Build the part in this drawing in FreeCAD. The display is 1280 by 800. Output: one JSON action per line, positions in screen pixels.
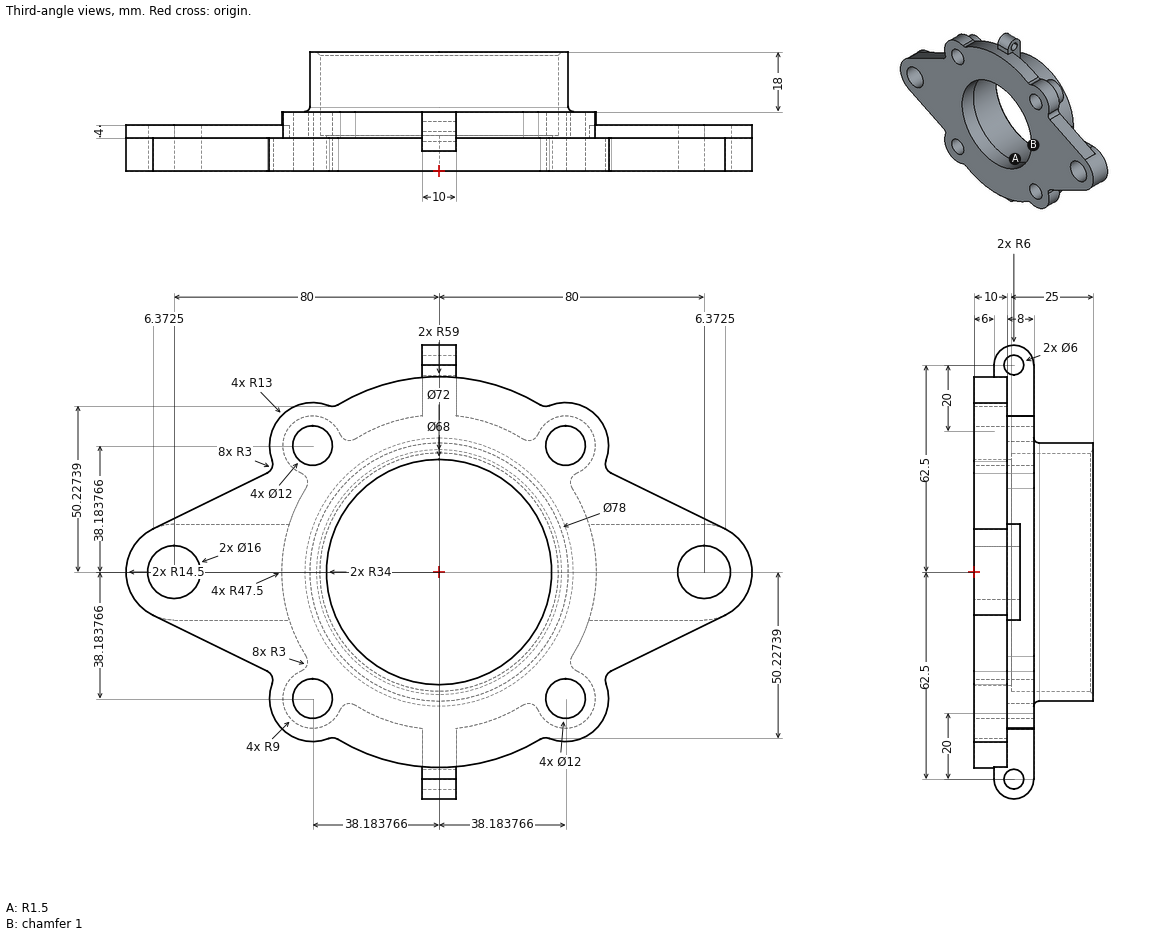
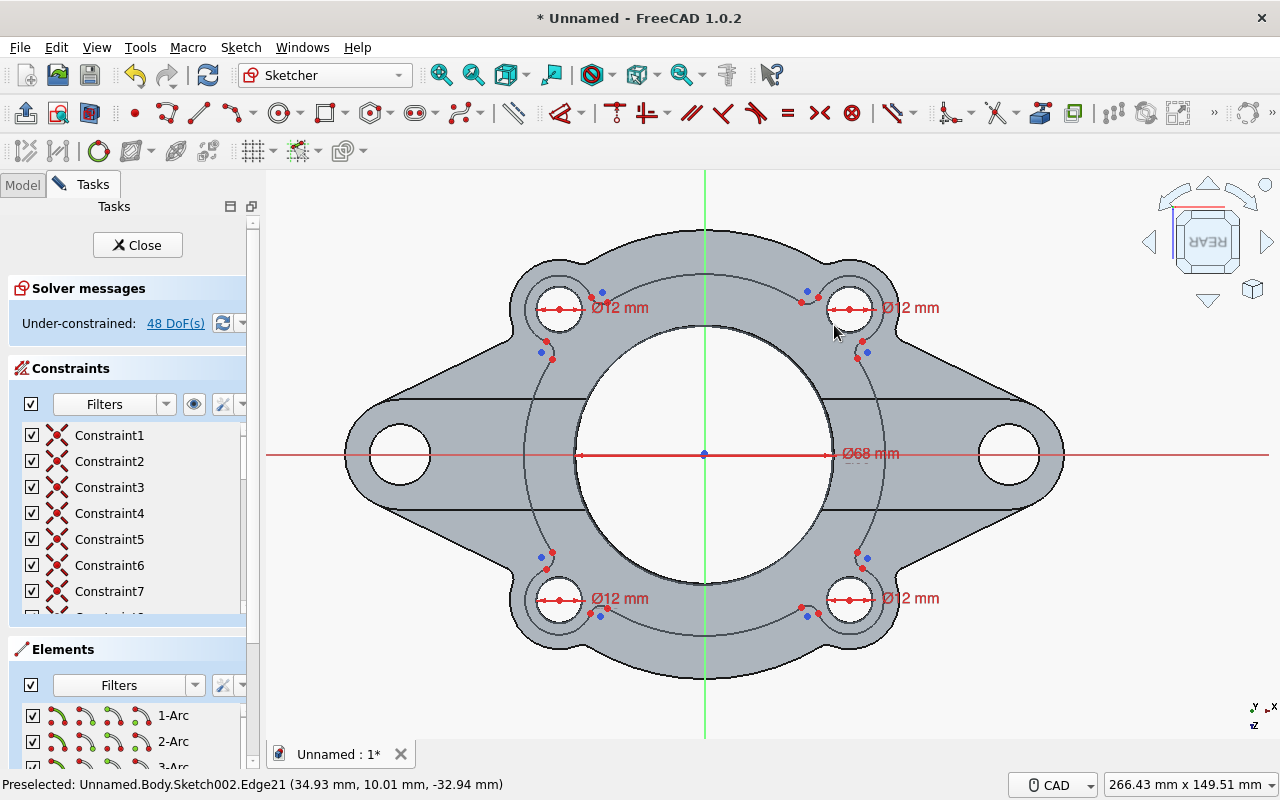
{"action": "left_click", "coordinate": [529, 415]}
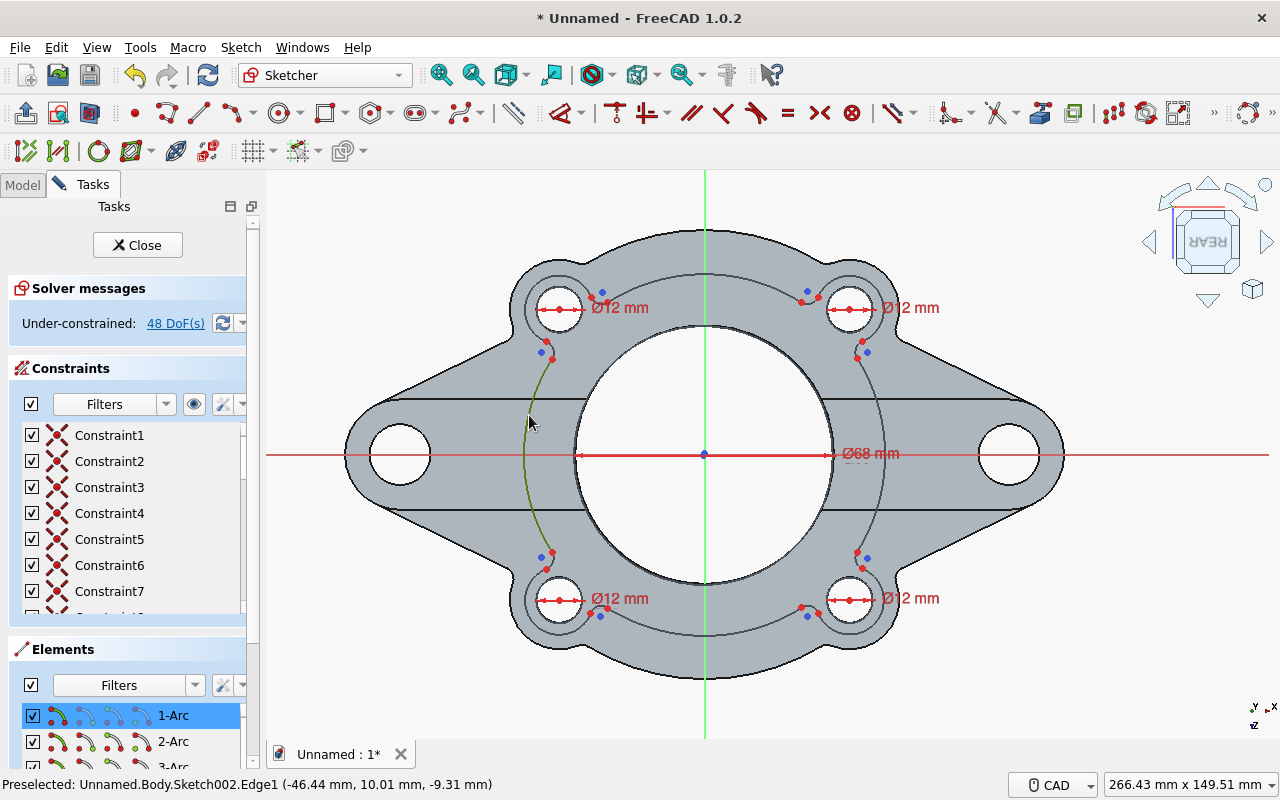
{"action": "scroll", "coordinate": [553, 562], "scroll_direction": "up", "scroll_amount": 2}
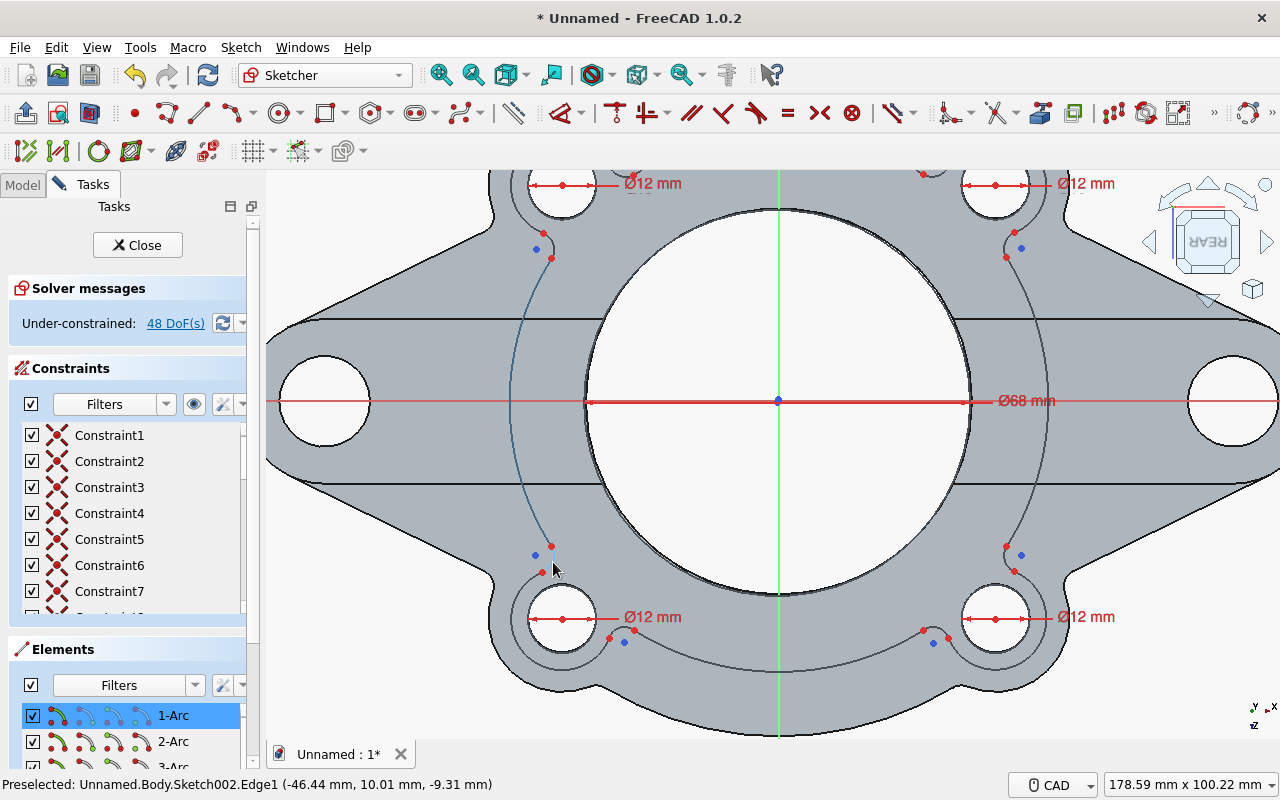
{"action": "left_click", "coordinate": [553, 562]}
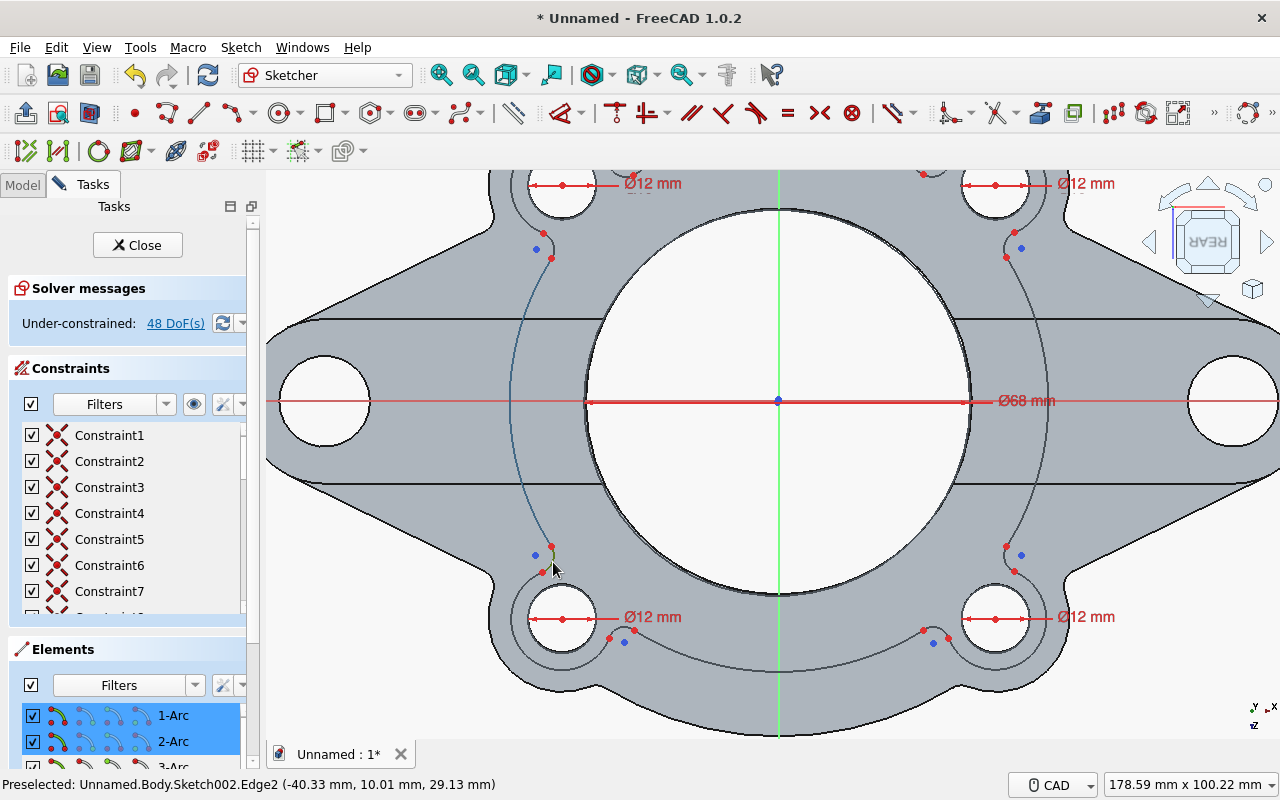
{"action": "left_click", "coordinate": [756, 114]}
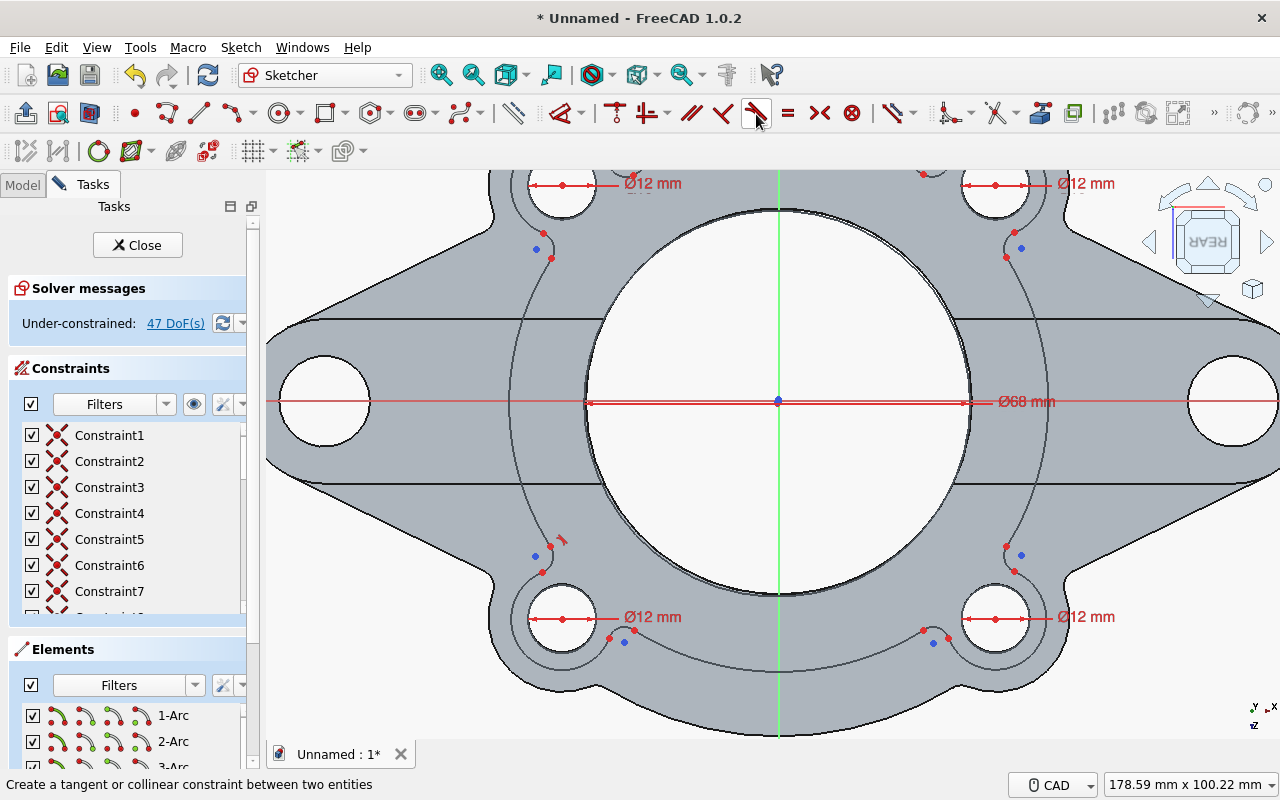
{"action": "left_click", "coordinate": [516, 342]}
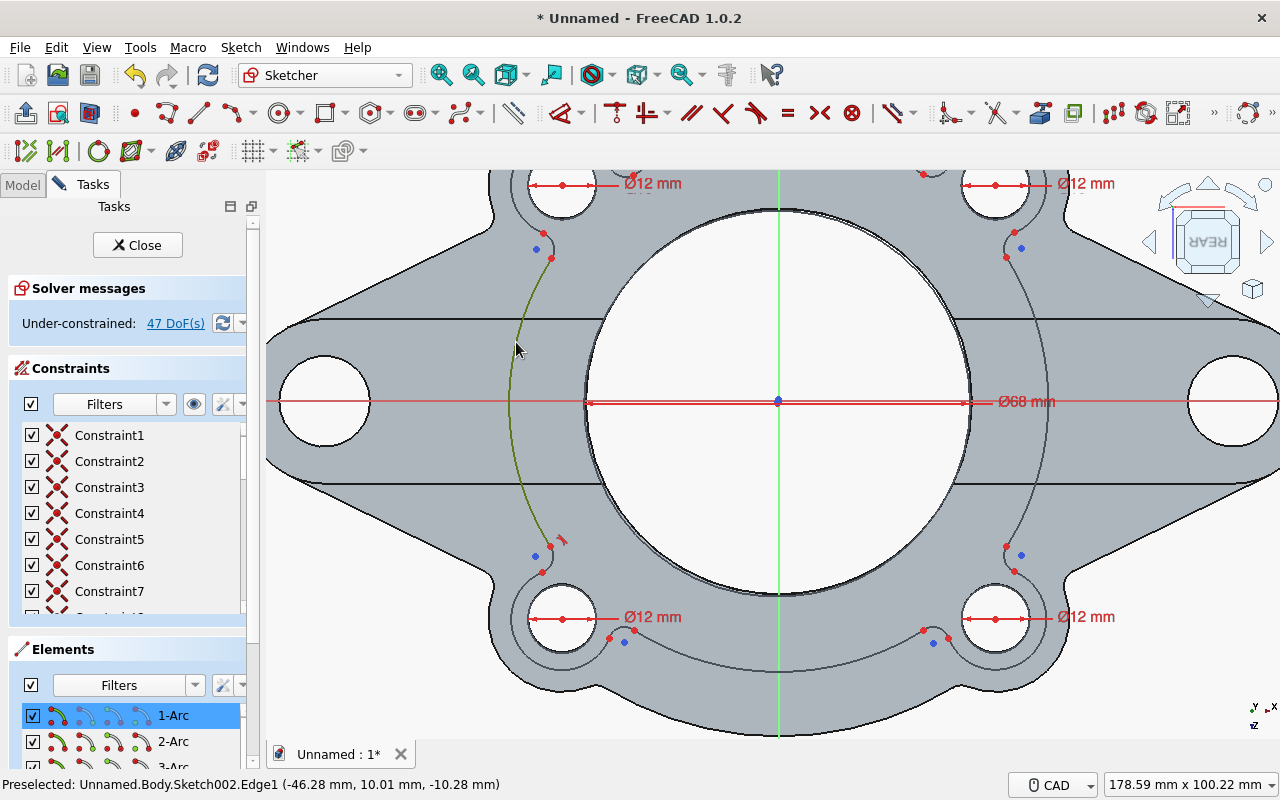
{"action": "scroll", "coordinate": [554, 250], "scroll_direction": "up", "scroll_amount": 3}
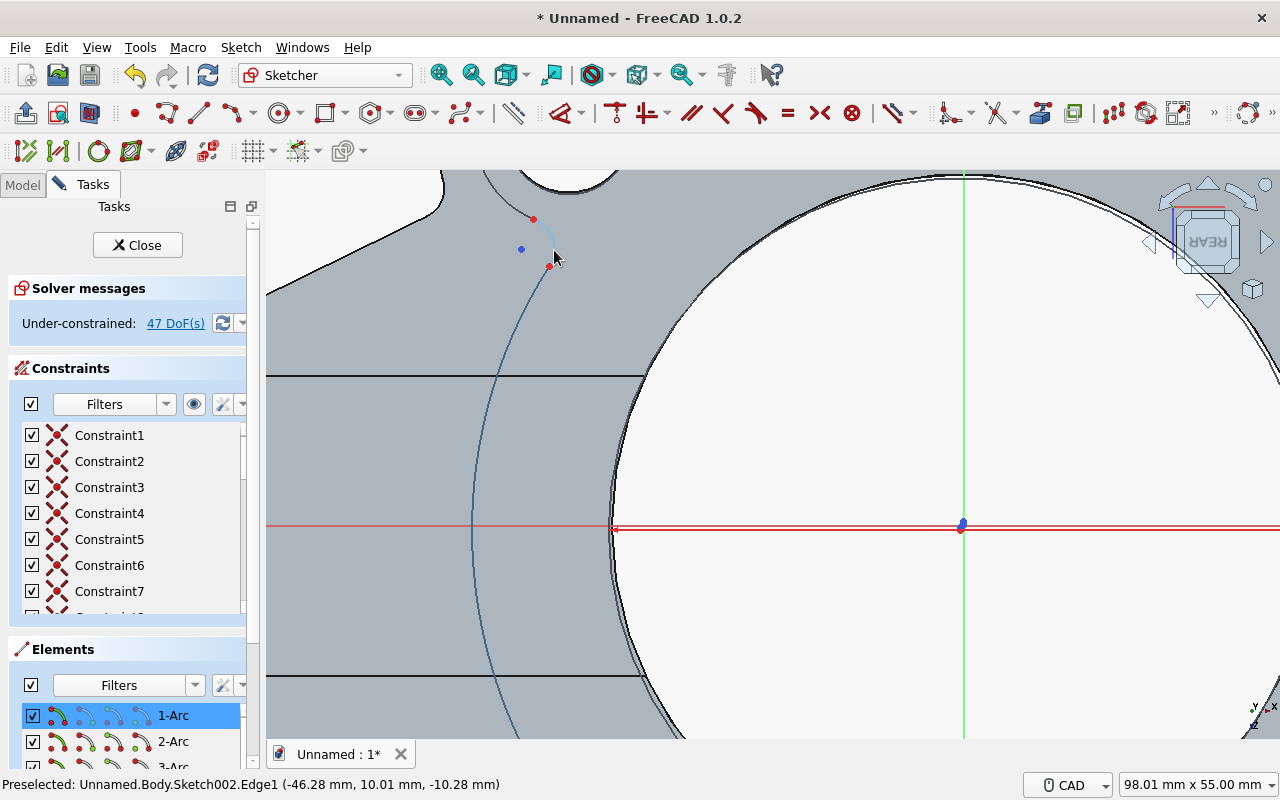
{"action": "left_click", "coordinate": [554, 250]}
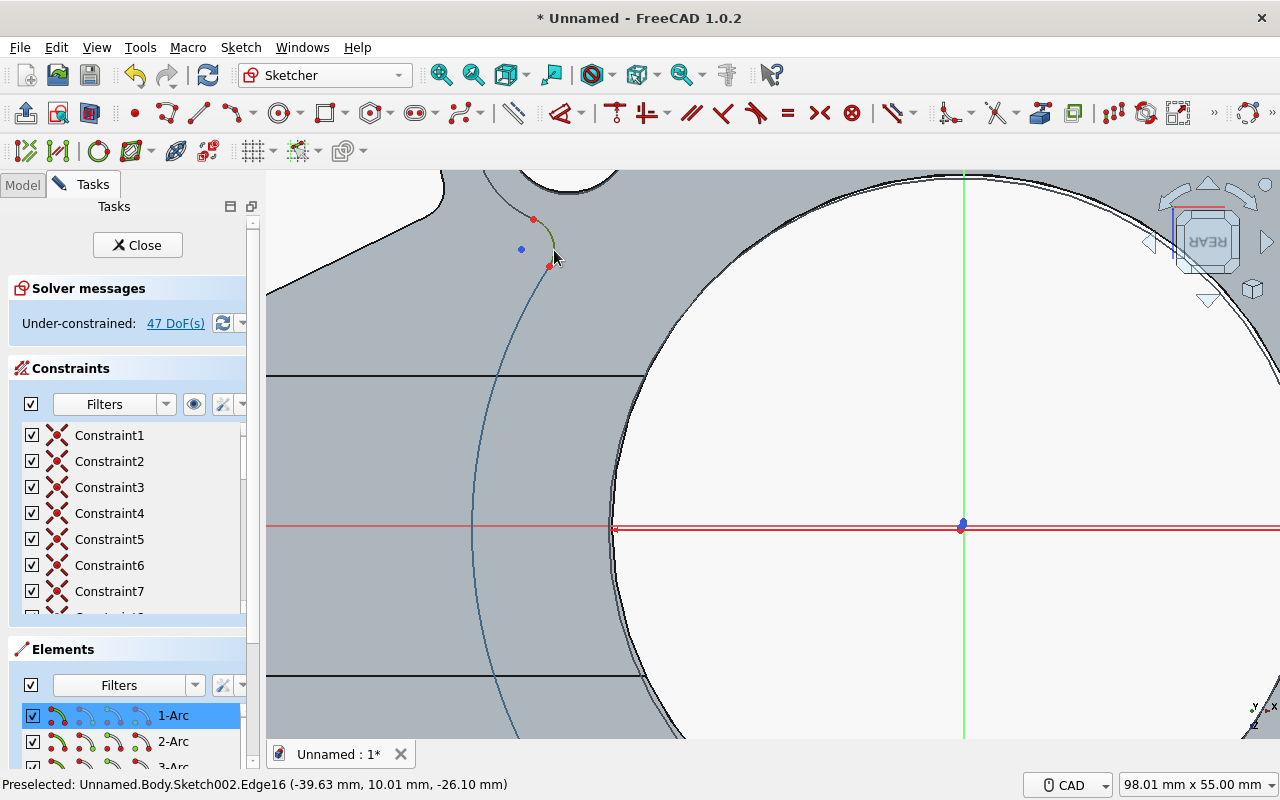
{"action": "left_click", "coordinate": [756, 114]}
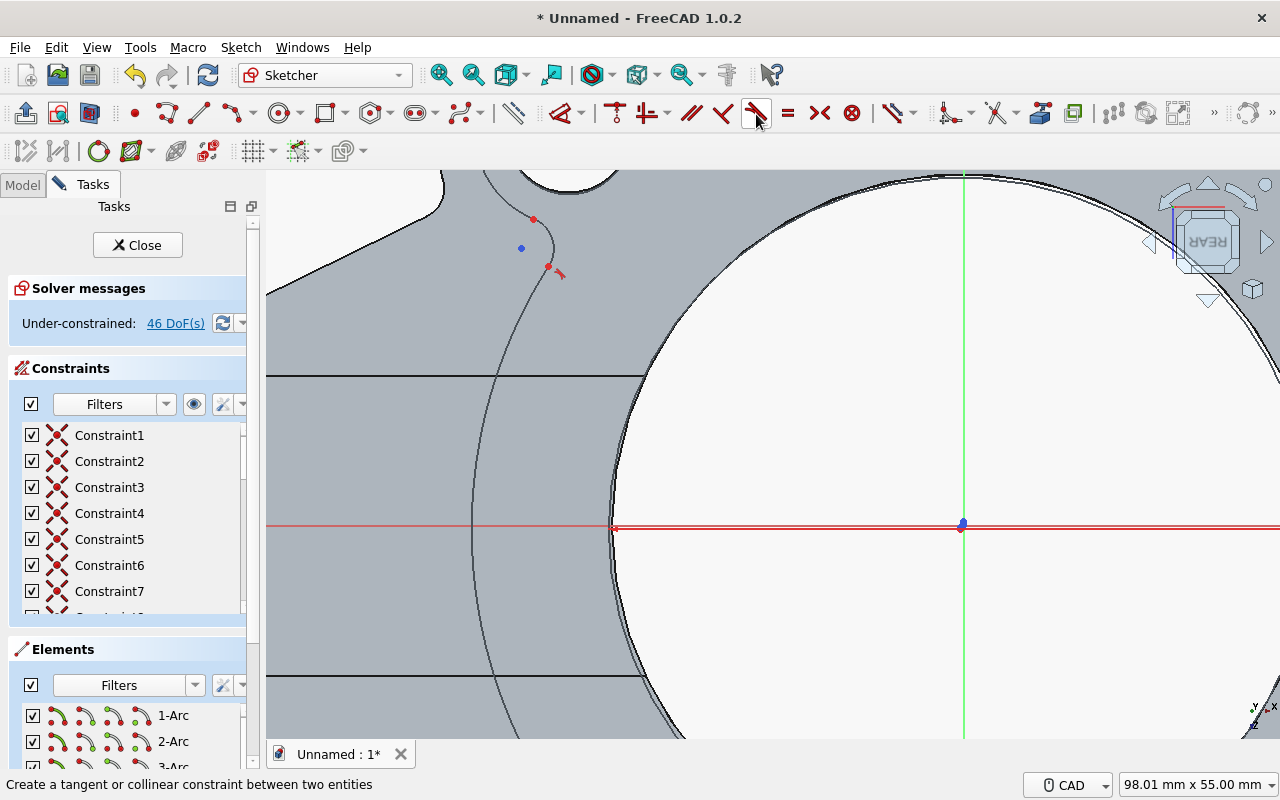
{"action": "scroll", "coordinate": [554, 413], "scroll_direction": "down", "scroll_amount": 5}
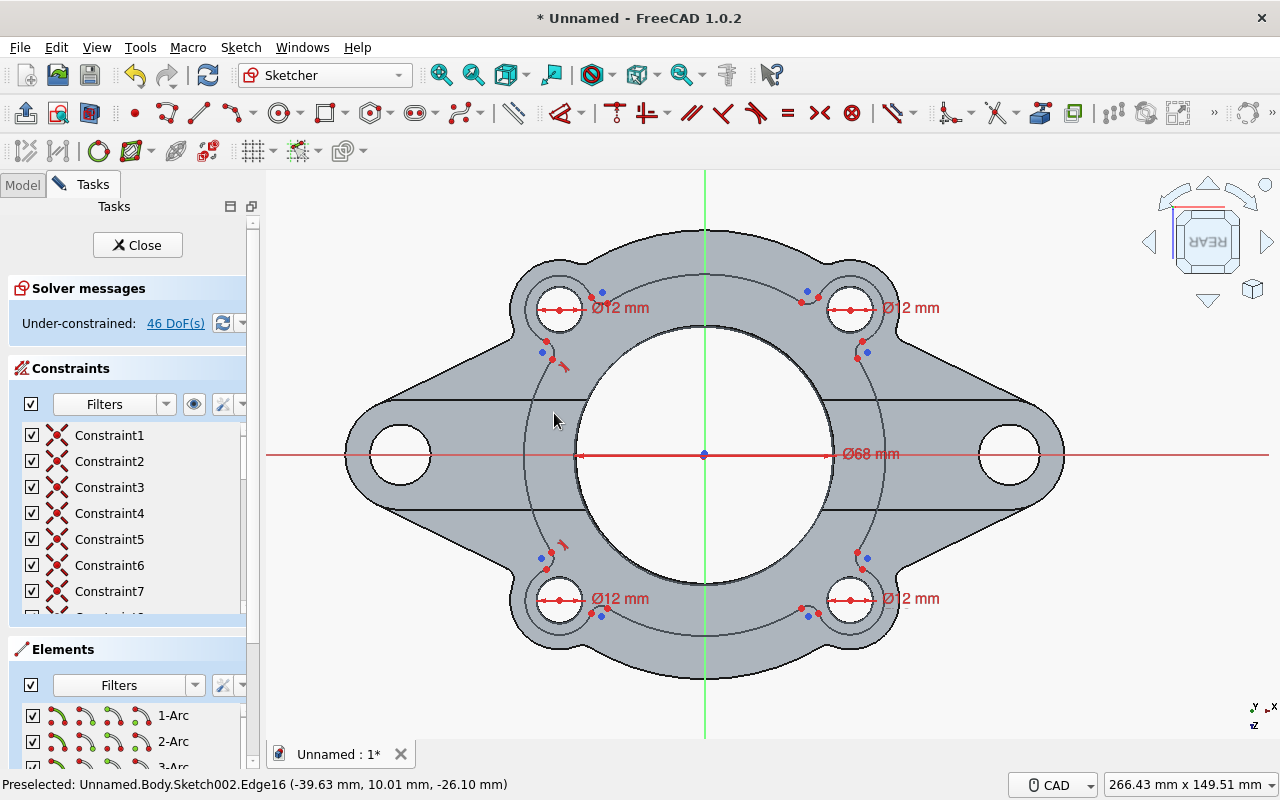
{"action": "scroll", "coordinate": [551, 566], "scroll_direction": "up", "scroll_amount": 5}